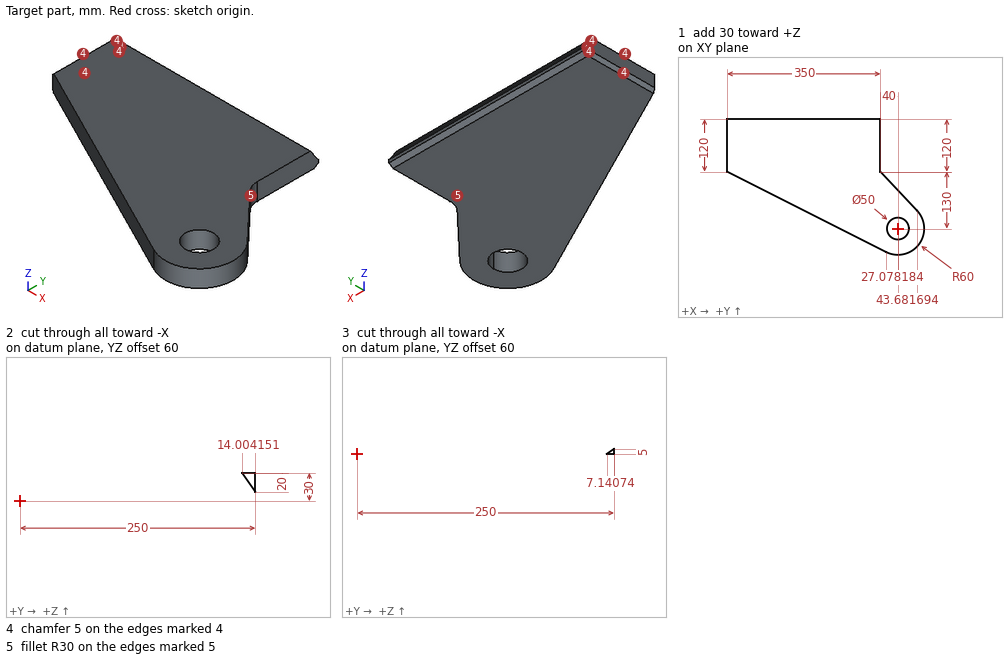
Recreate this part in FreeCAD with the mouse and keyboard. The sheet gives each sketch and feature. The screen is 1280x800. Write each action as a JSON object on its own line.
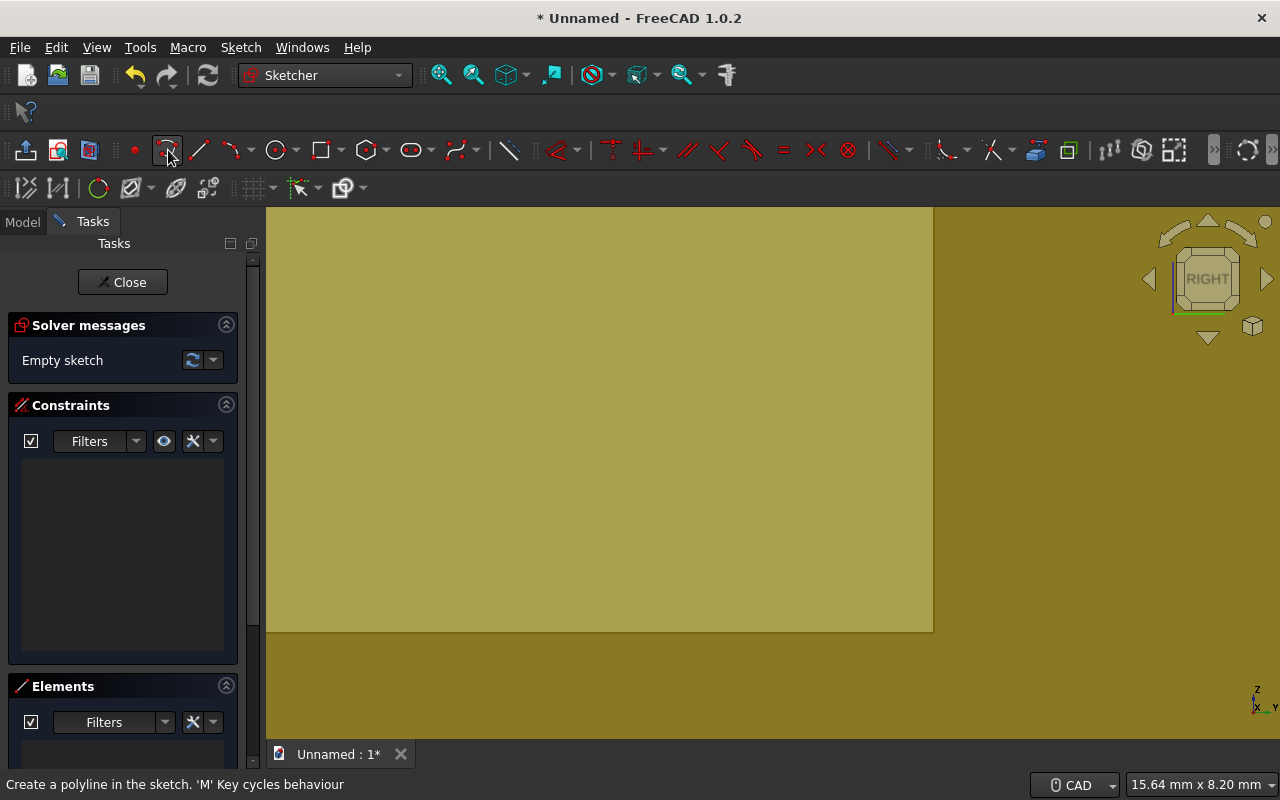
{"action": "left_click", "coordinate": [471, 633]}
{"action": "left_click", "coordinate": [934, 624]}
{"action": "left_click", "coordinate": [934, 309]}
{"action": "left_click", "coordinate": [471, 634]}
{"action": "key", "text": "Escape"}
{"action": "key", "text": "Escape"}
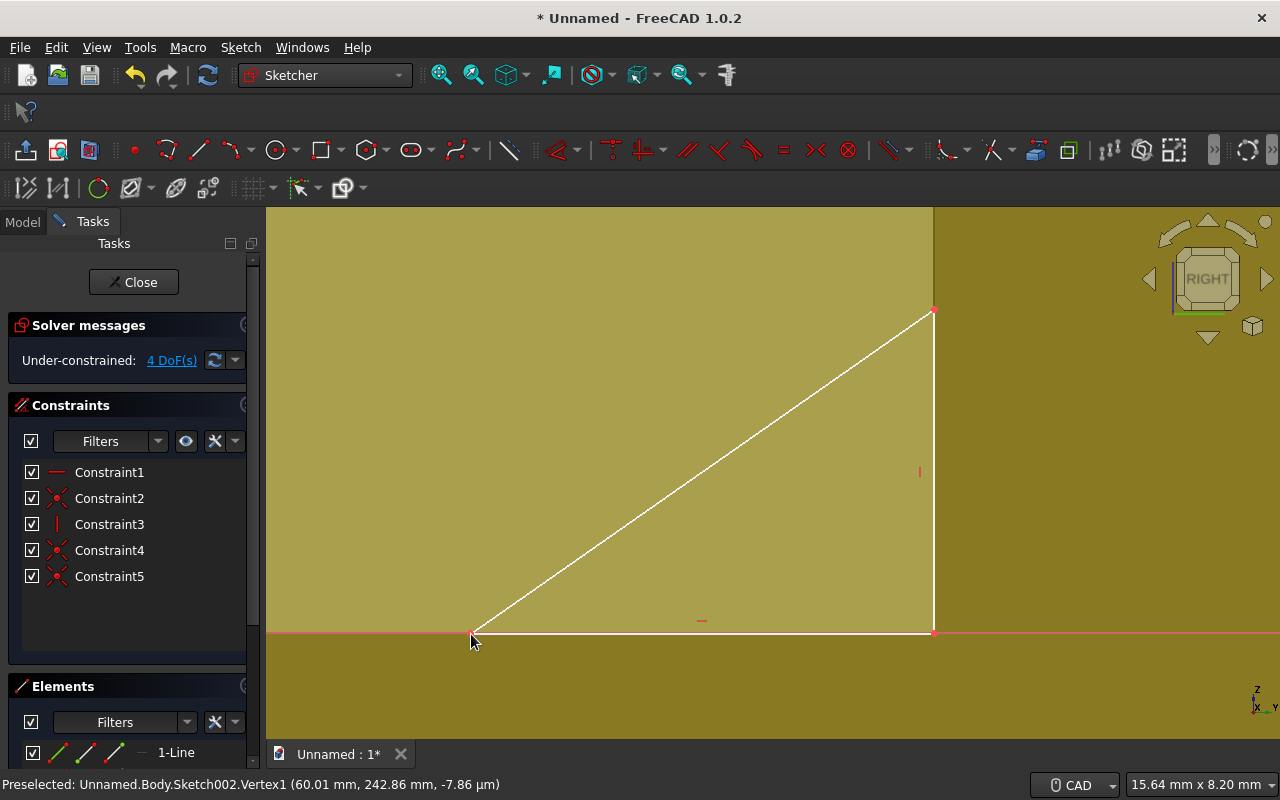
{"action": "left_click", "coordinate": [471, 634]}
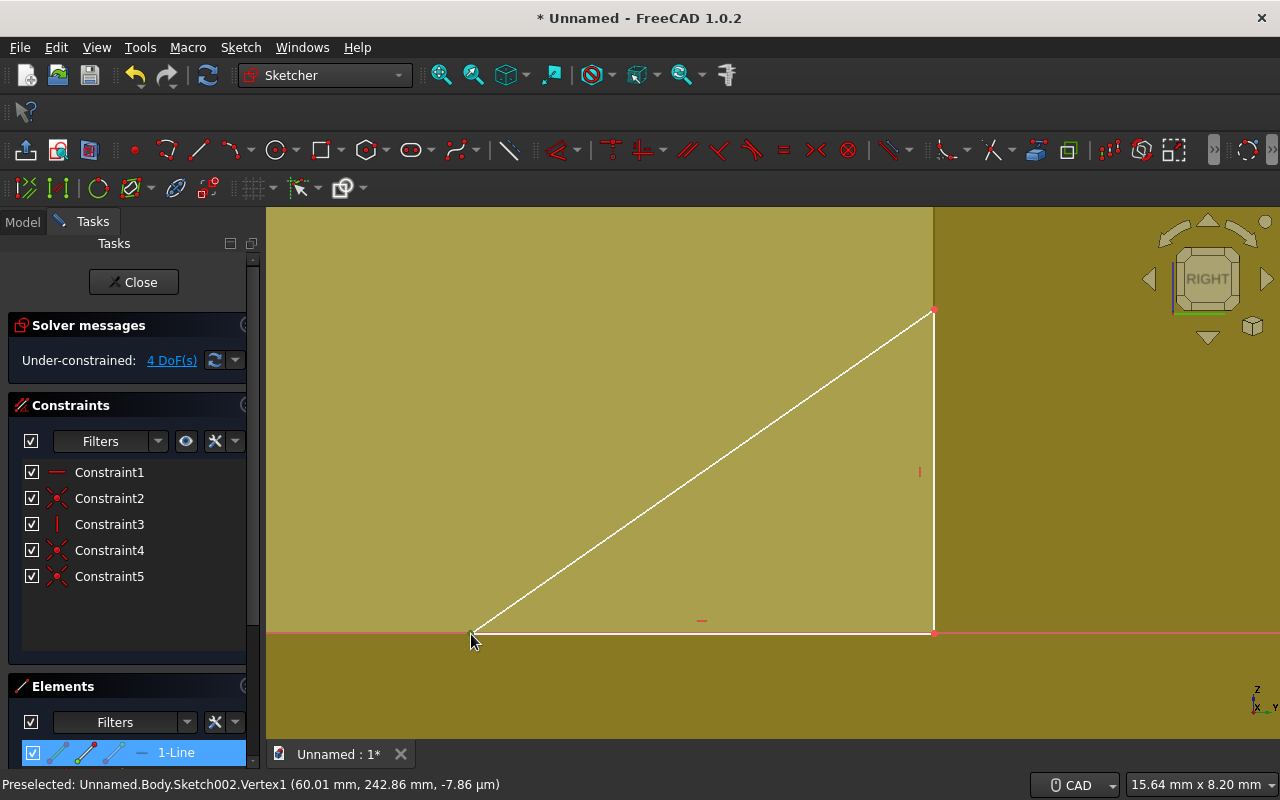
{"action": "left_click", "coordinate": [353, 633]}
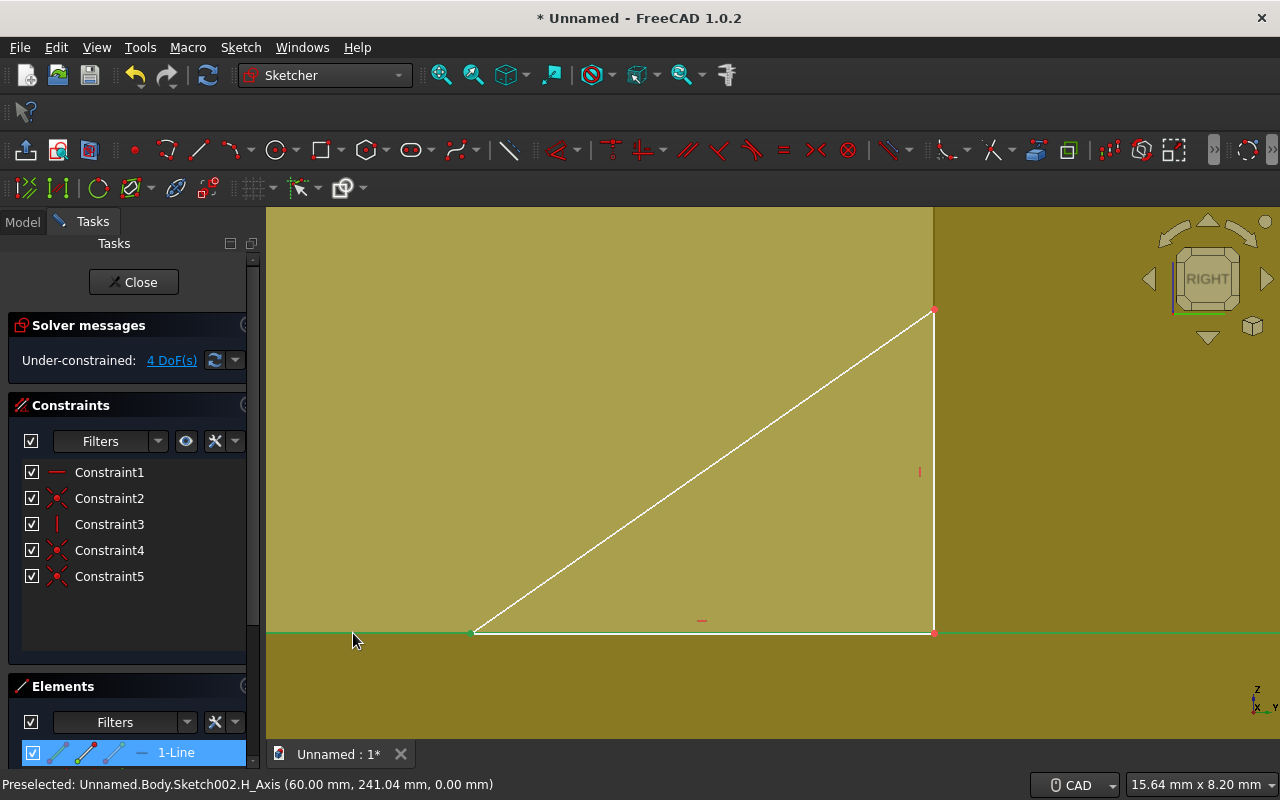
{"action": "key", "text": "c"}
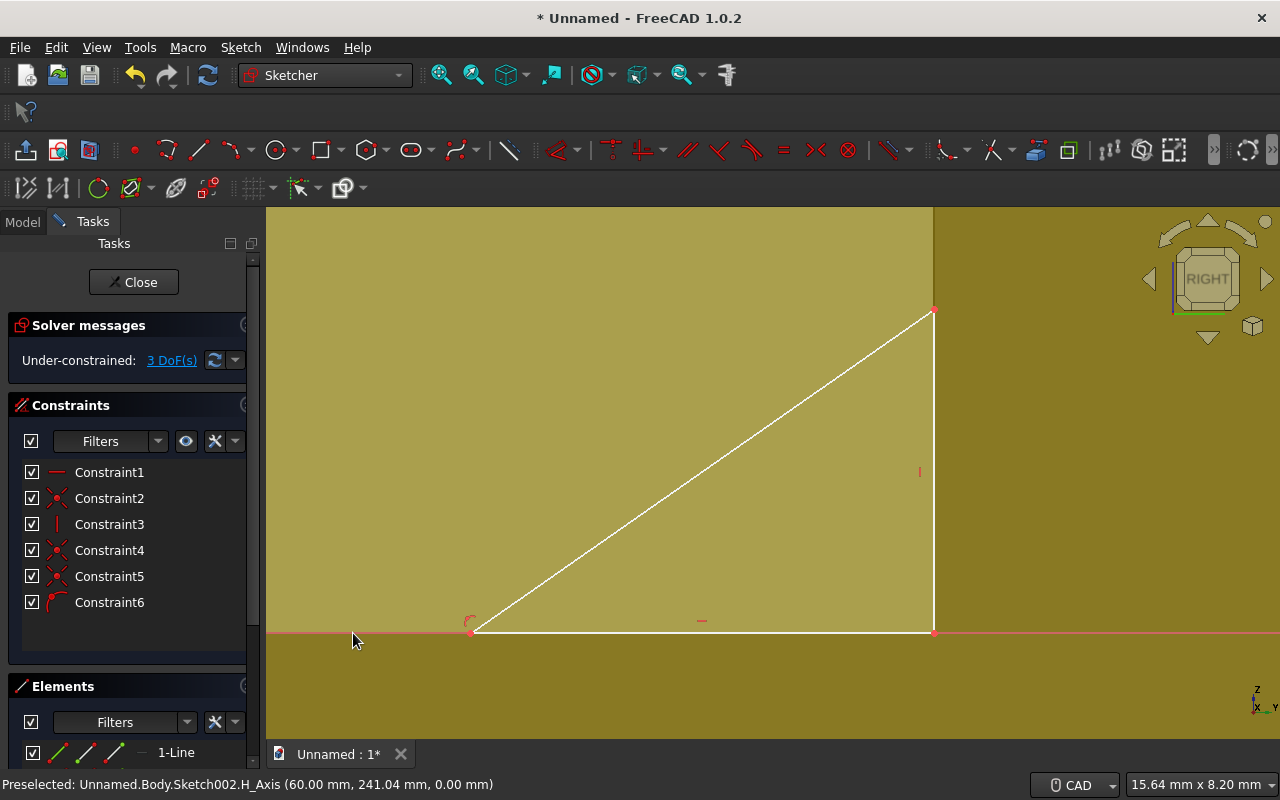
{"action": "left_click", "coordinate": [556, 150]}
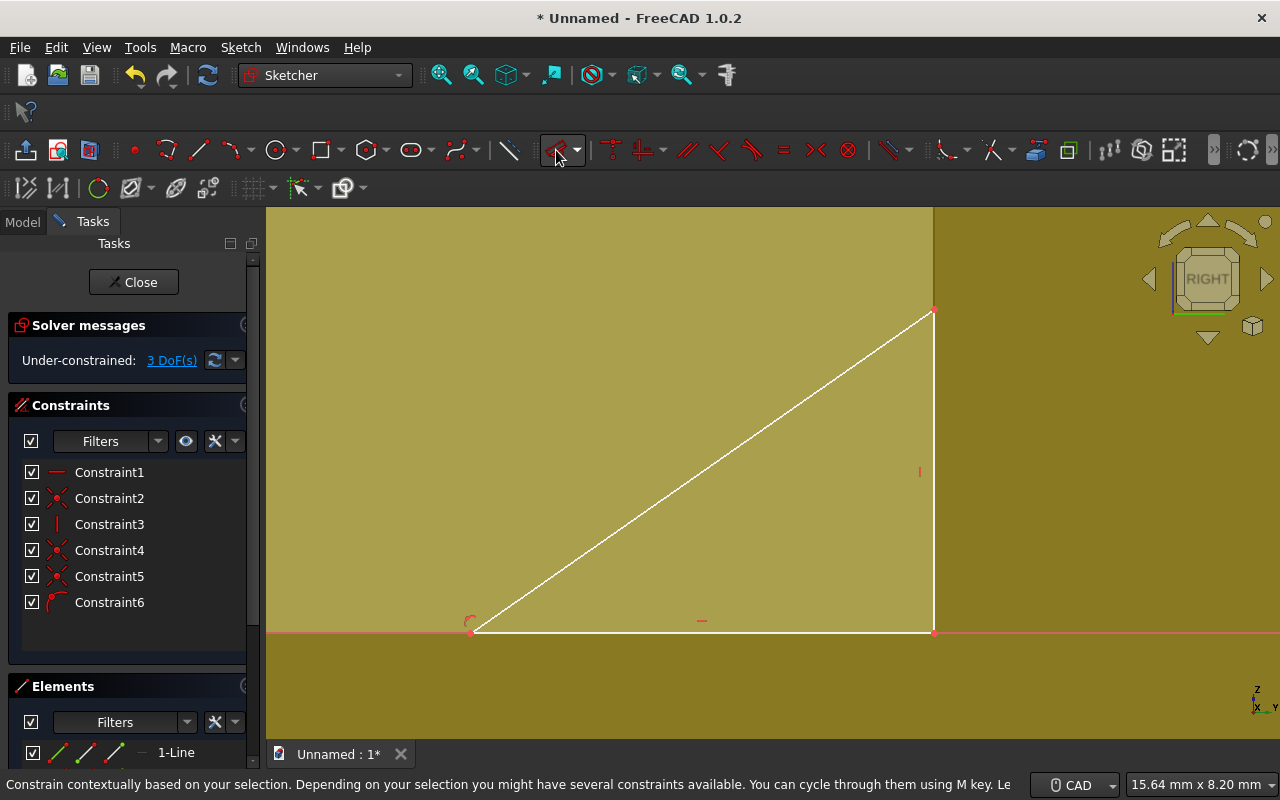
{"action": "left_click", "coordinate": [934, 536]}
{"action": "left_click", "coordinate": [968, 472]}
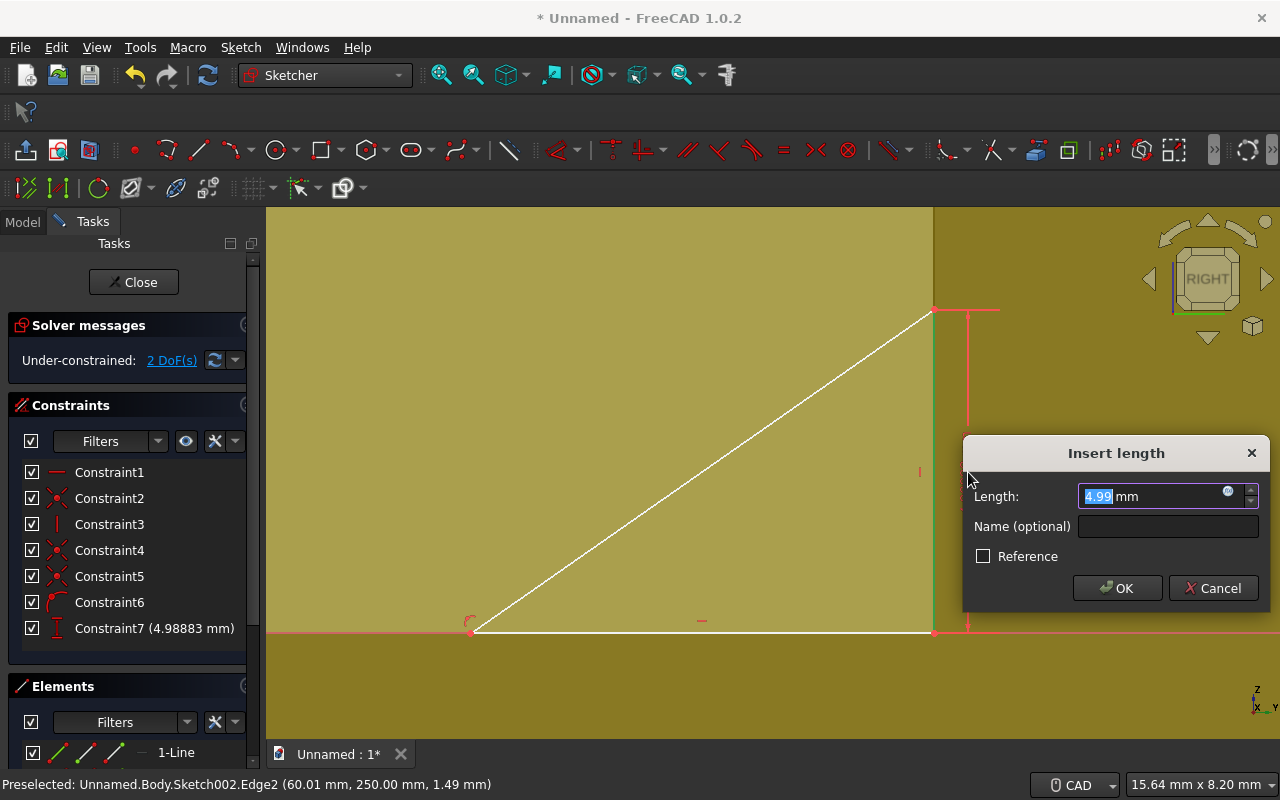
{"action": "type", "text": "5"}
{"action": "key", "text": "Return"}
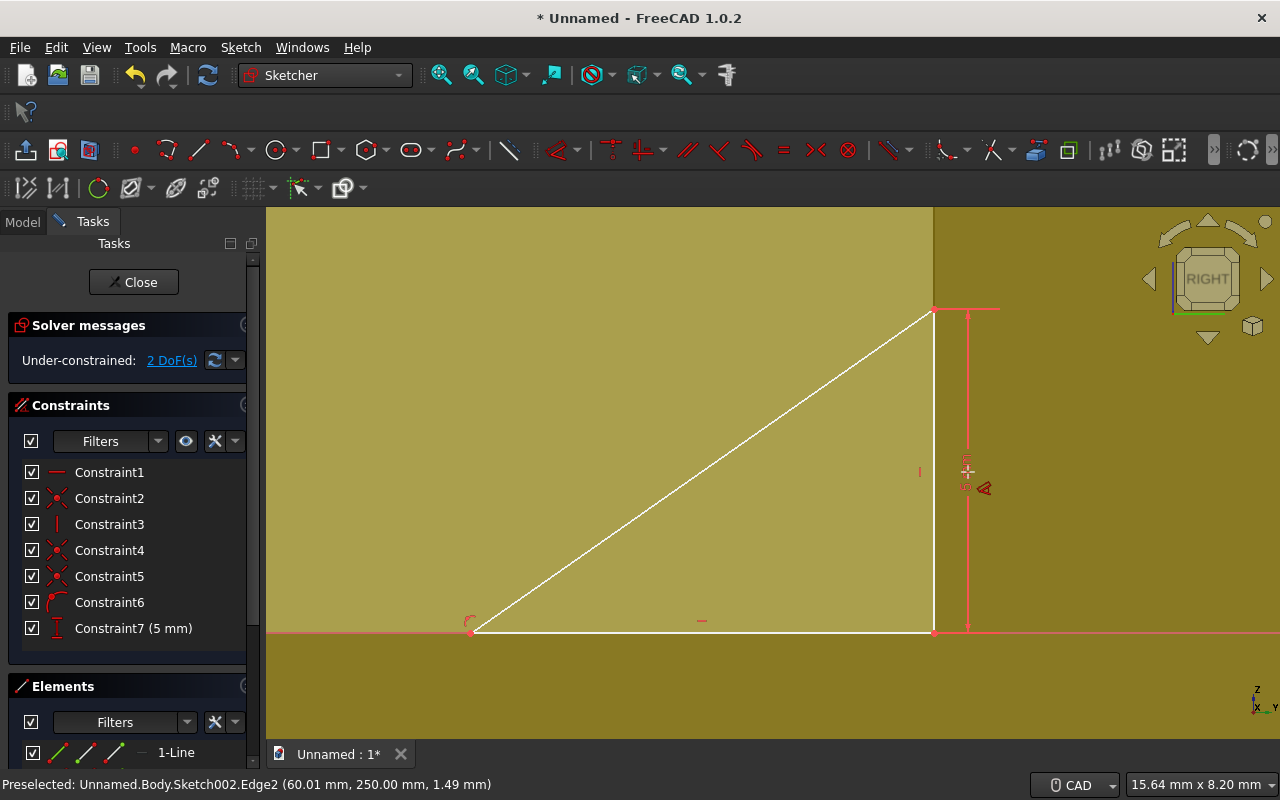
{"action": "left_click", "coordinate": [934, 633]}
{"action": "left_click", "coordinate": [614, 667]}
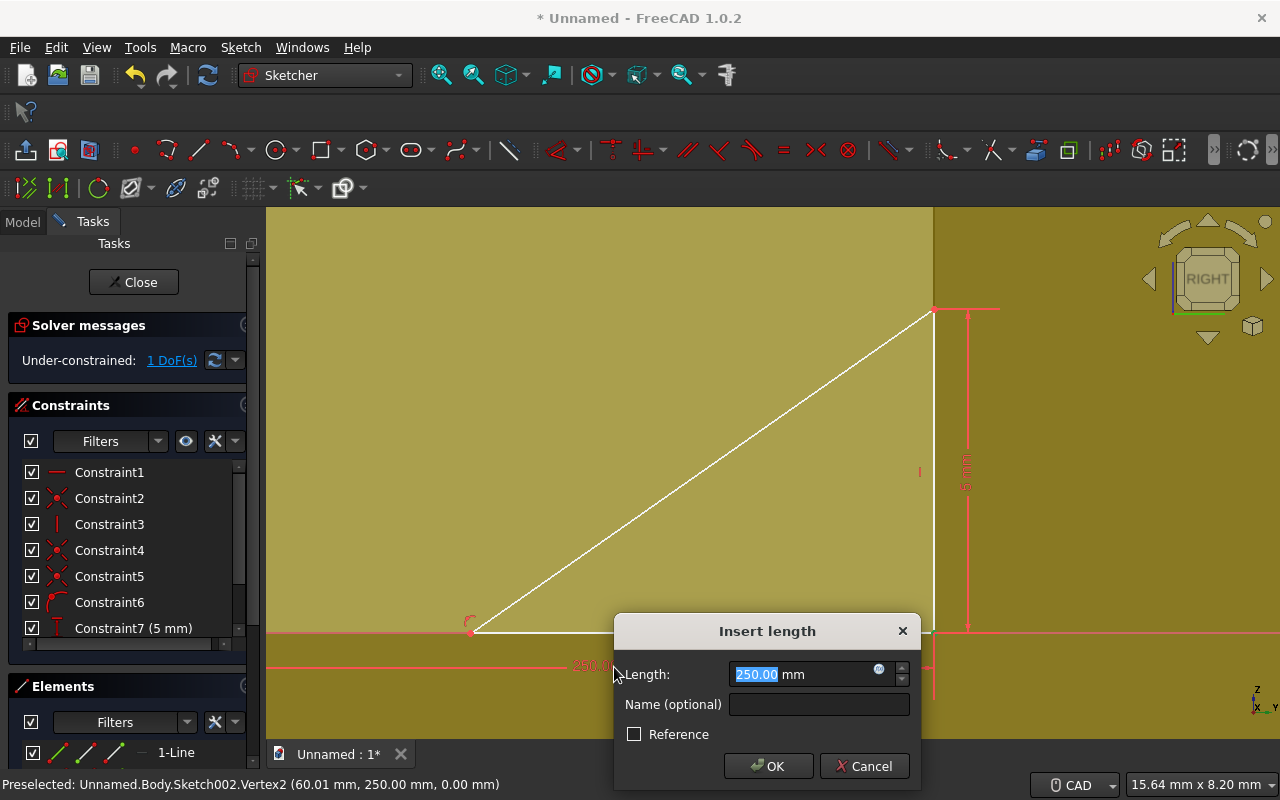
{"action": "type", "text": "250"}
{"action": "key", "text": "Return"}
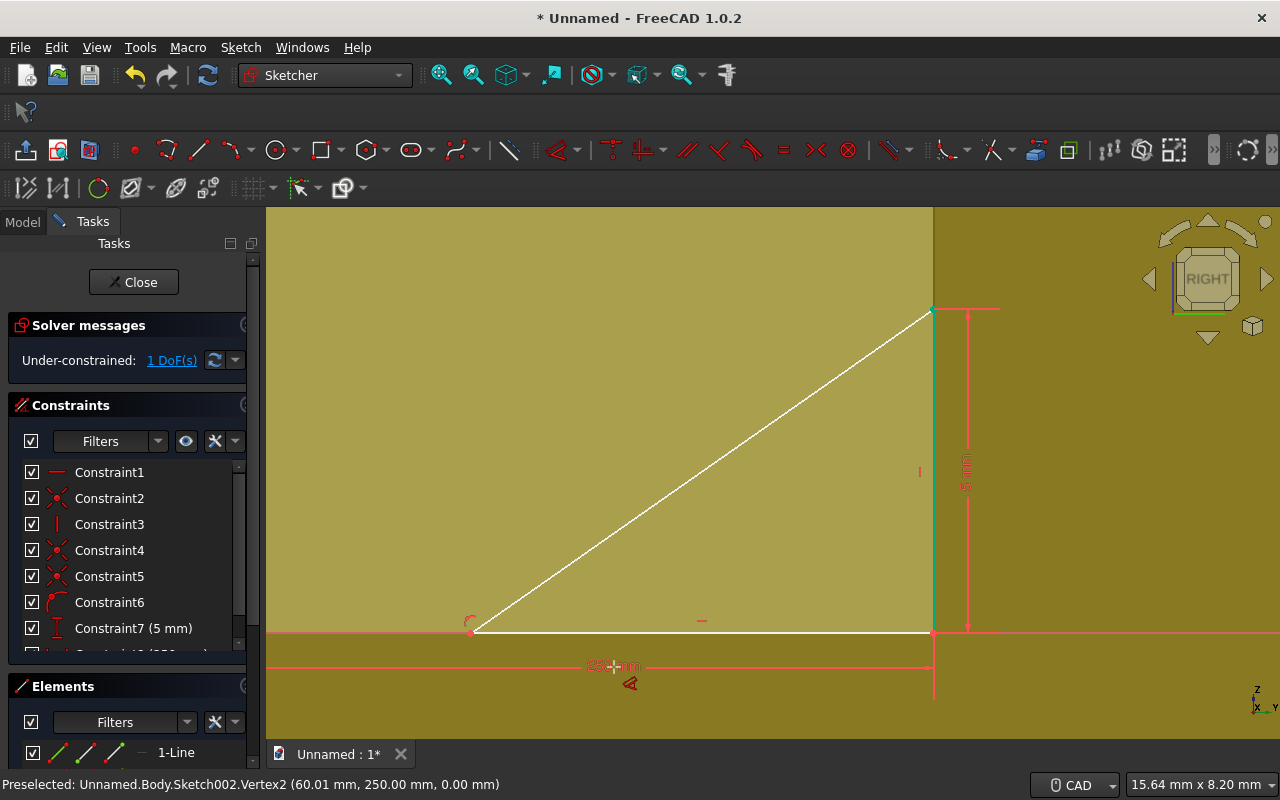
{"action": "left_click", "coordinate": [610, 633]}
{"action": "left_click", "coordinate": [702, 667]}